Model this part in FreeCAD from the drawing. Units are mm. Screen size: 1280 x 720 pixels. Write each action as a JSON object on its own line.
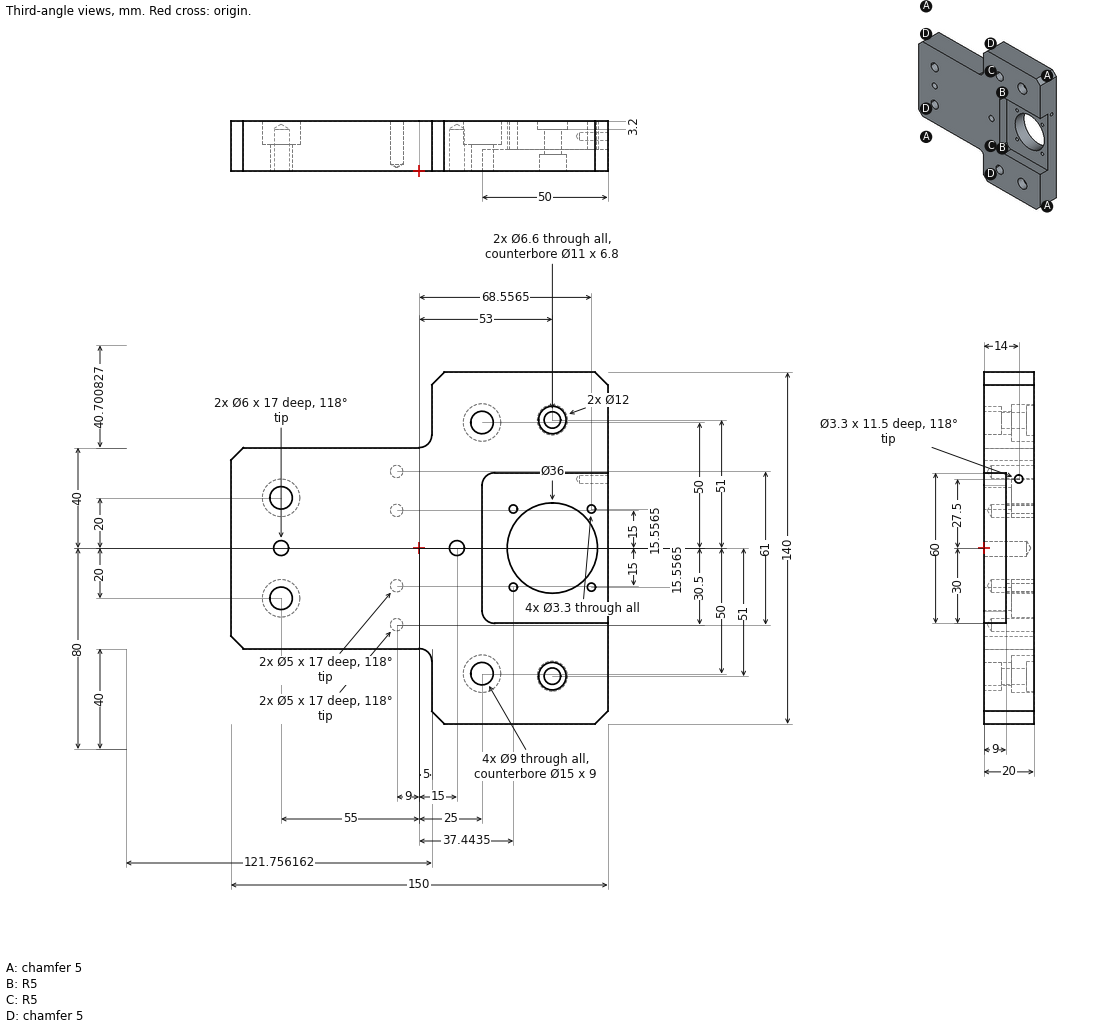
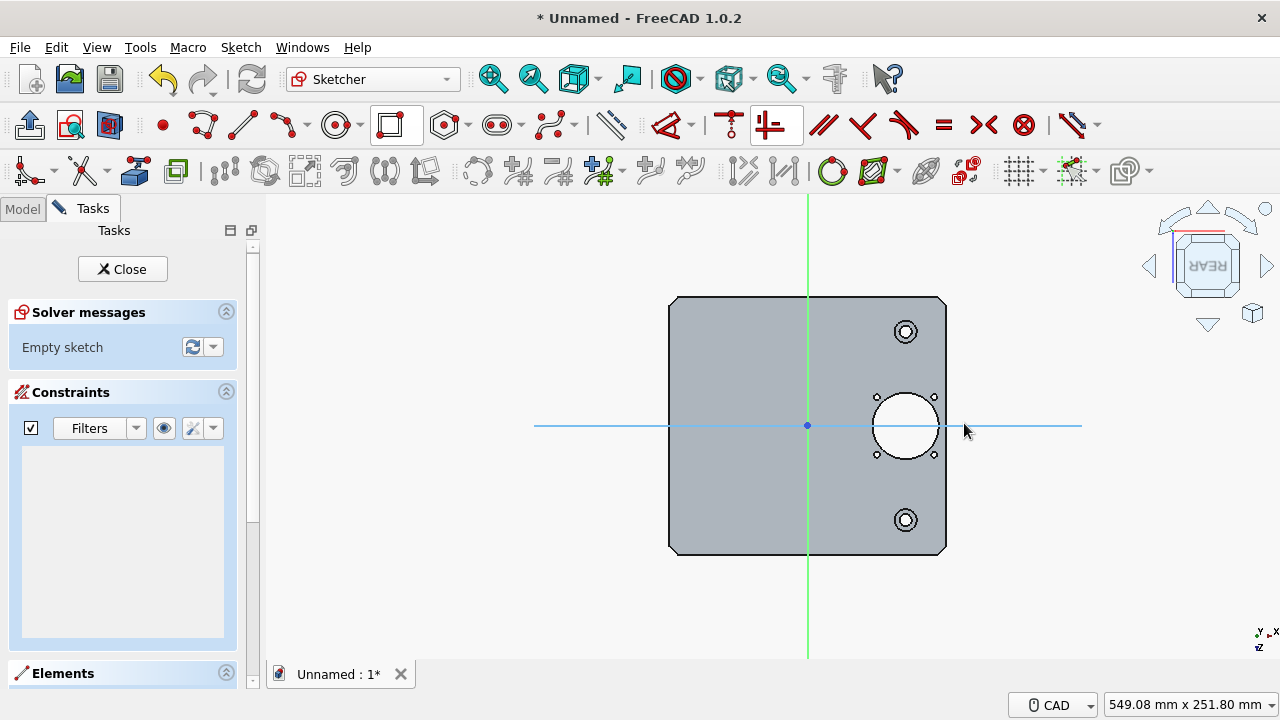
{"action": "left_click", "coordinate": [390, 126]}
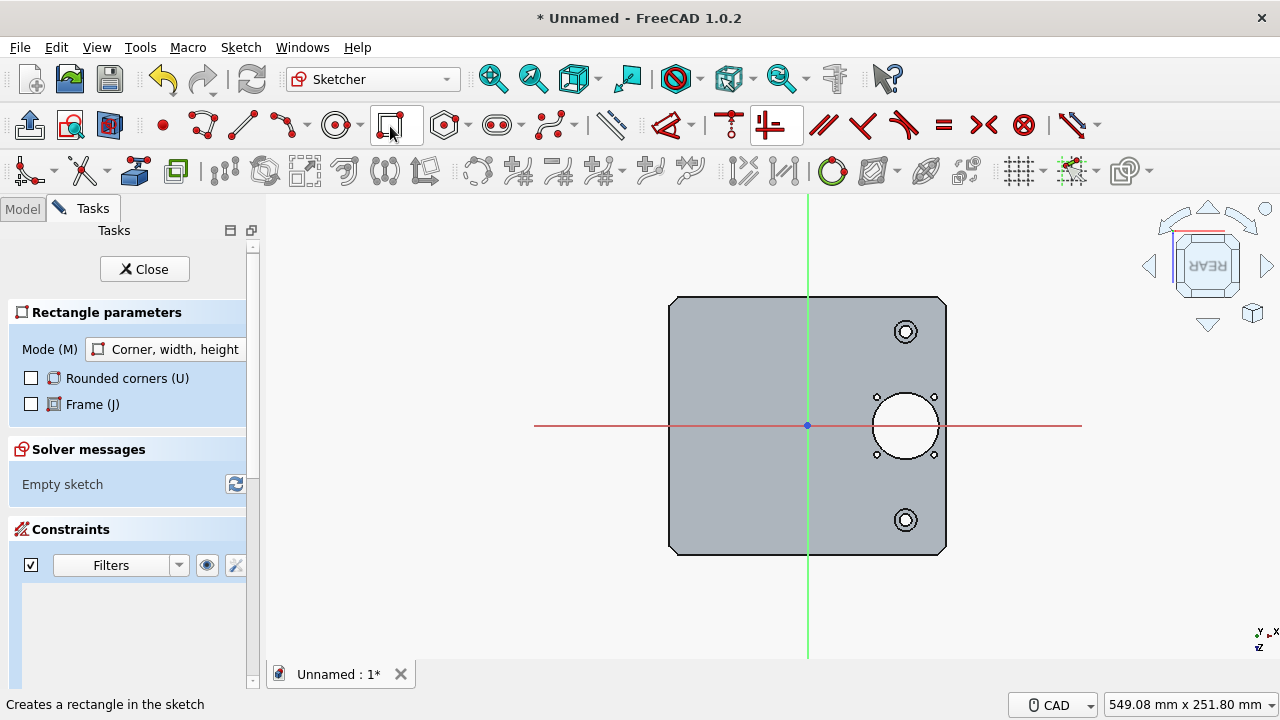
{"action": "left_click", "coordinate": [592, 278]}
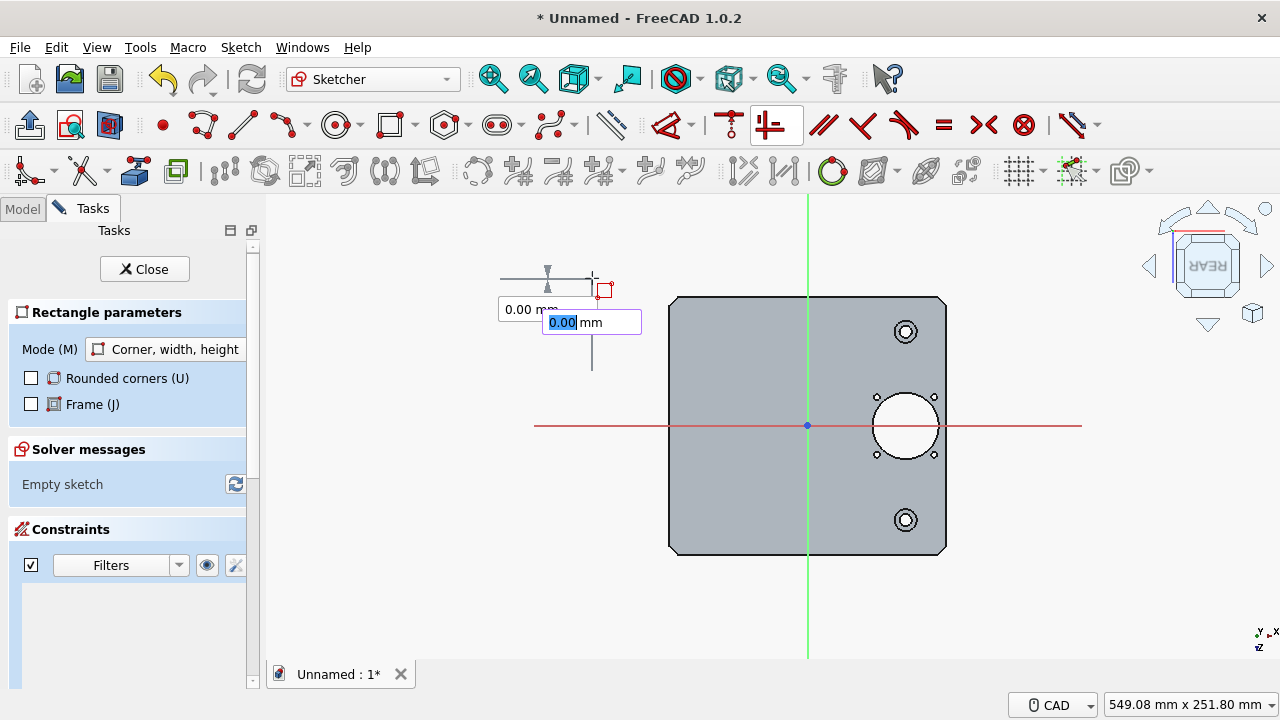
{"action": "scroll", "coordinate": [817, 352], "scroll_direction": "up", "scroll_amount": 3}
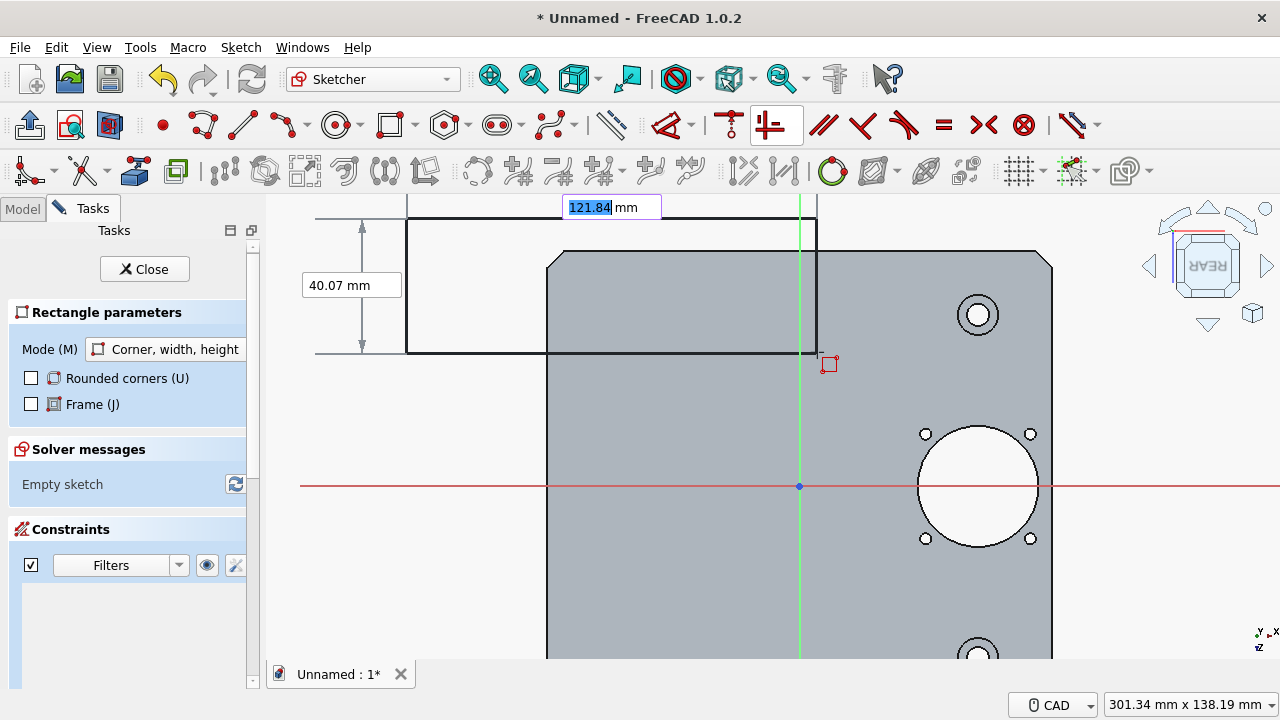
{"action": "left_click", "coordinate": [817, 352]}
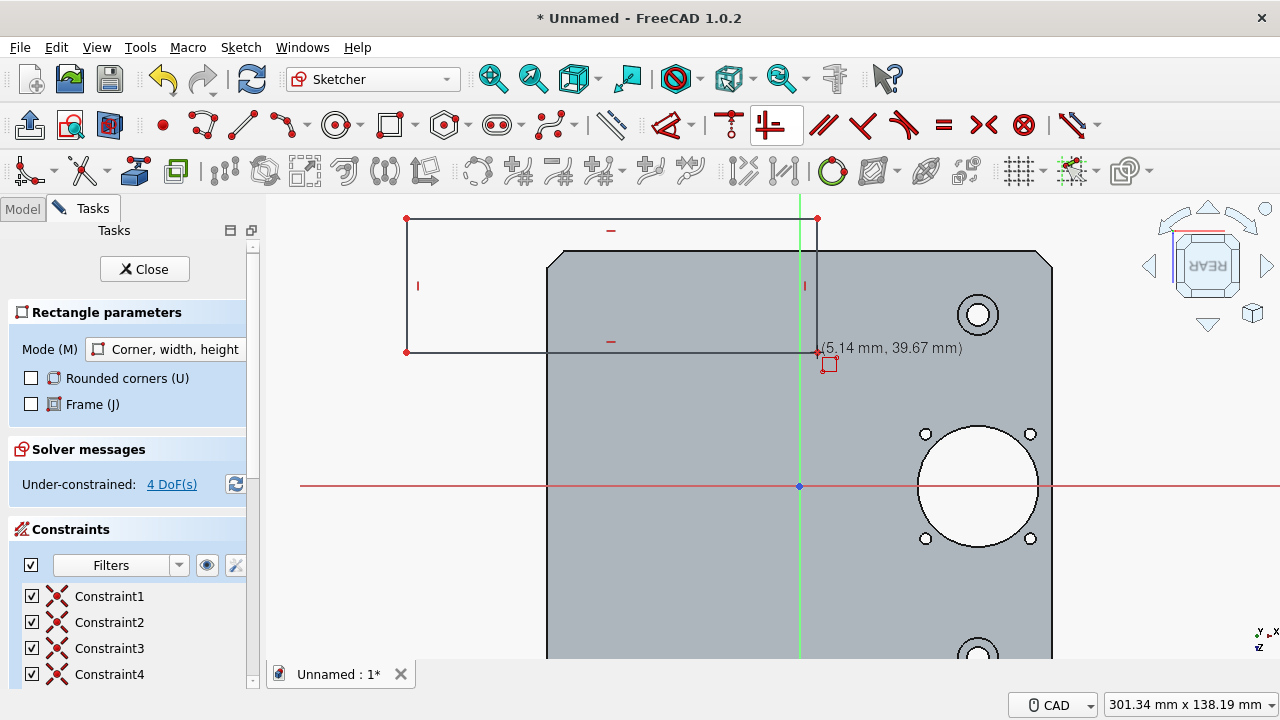
{"action": "left_click", "coordinate": [407, 621]}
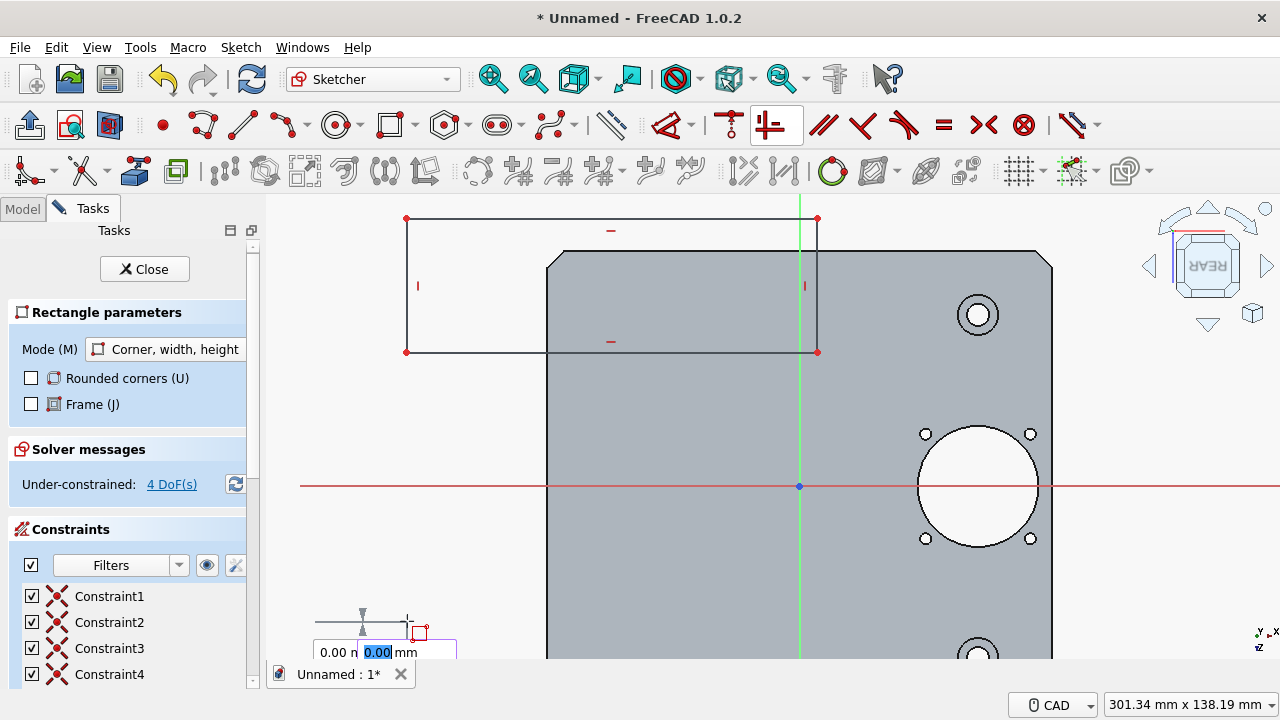
{"action": "scroll", "coordinate": [817, 352], "scroll_direction": "down", "scroll_amount": 3}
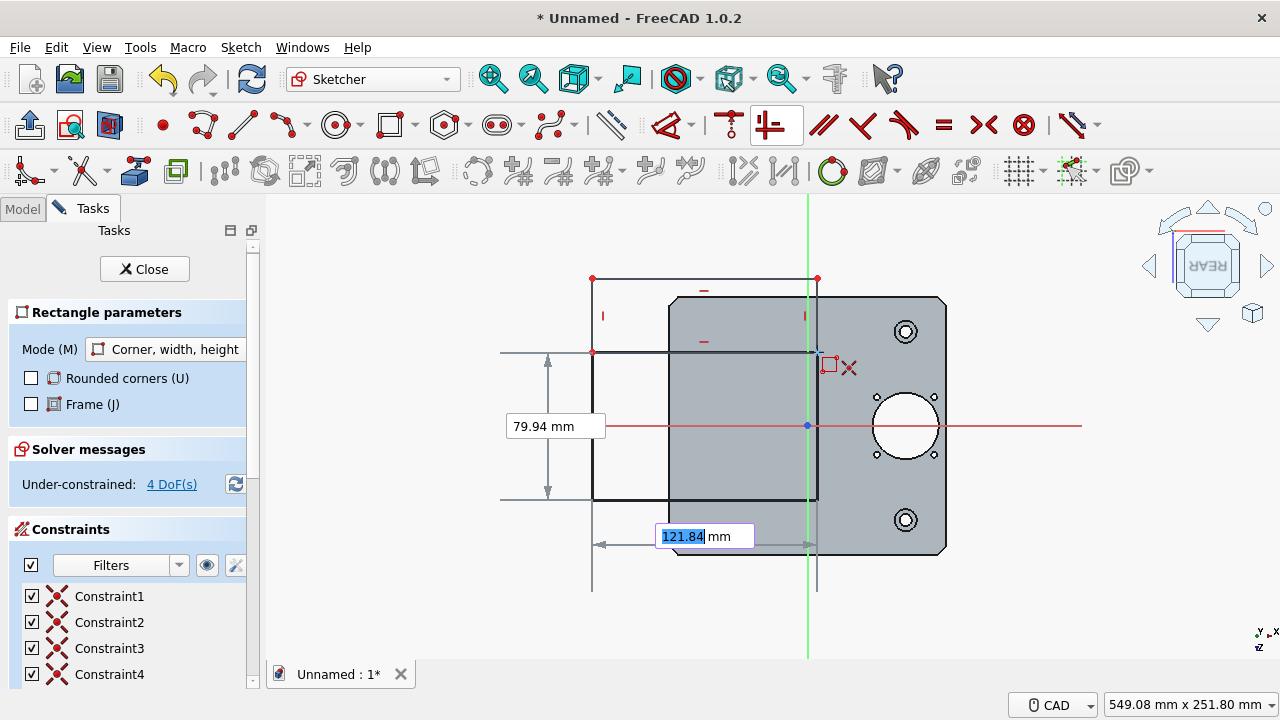
{"action": "scroll", "coordinate": [817, 575], "scroll_direction": "up", "scroll_amount": 3}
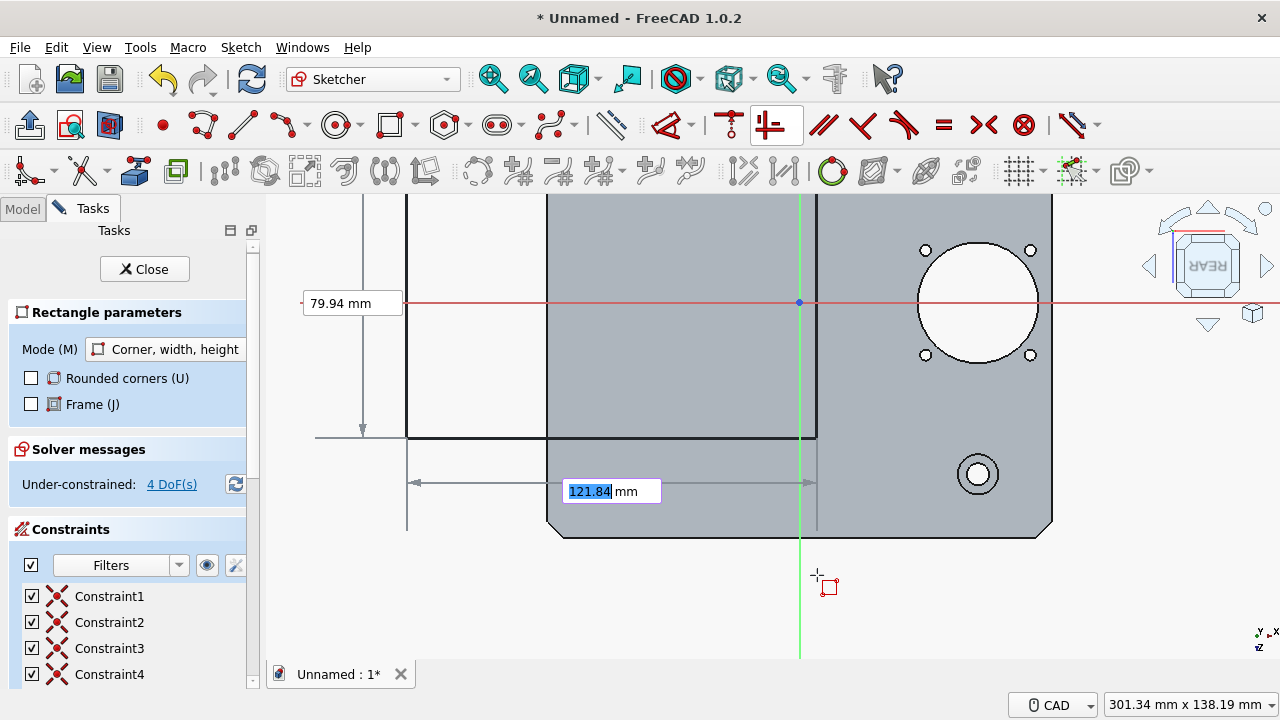
{"action": "left_click", "coordinate": [817, 574]}
{"action": "key", "text": "Escape"}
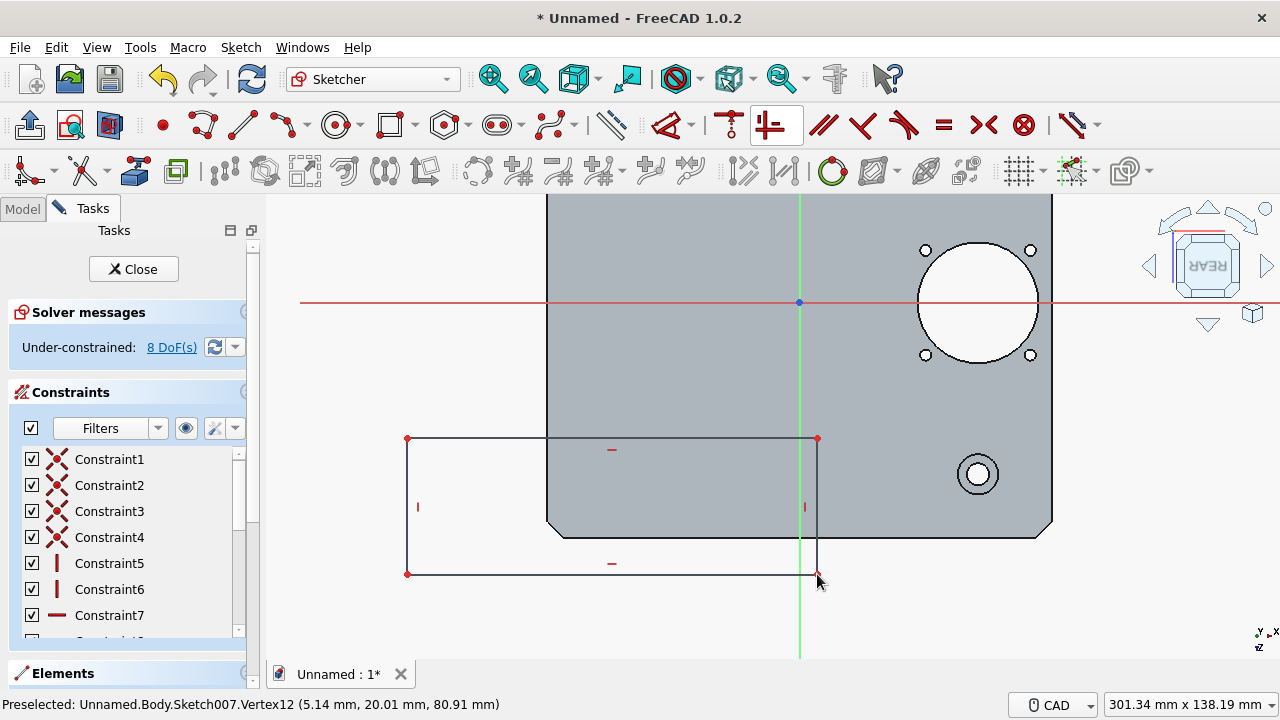
{"action": "left_click", "coordinate": [666, 126]}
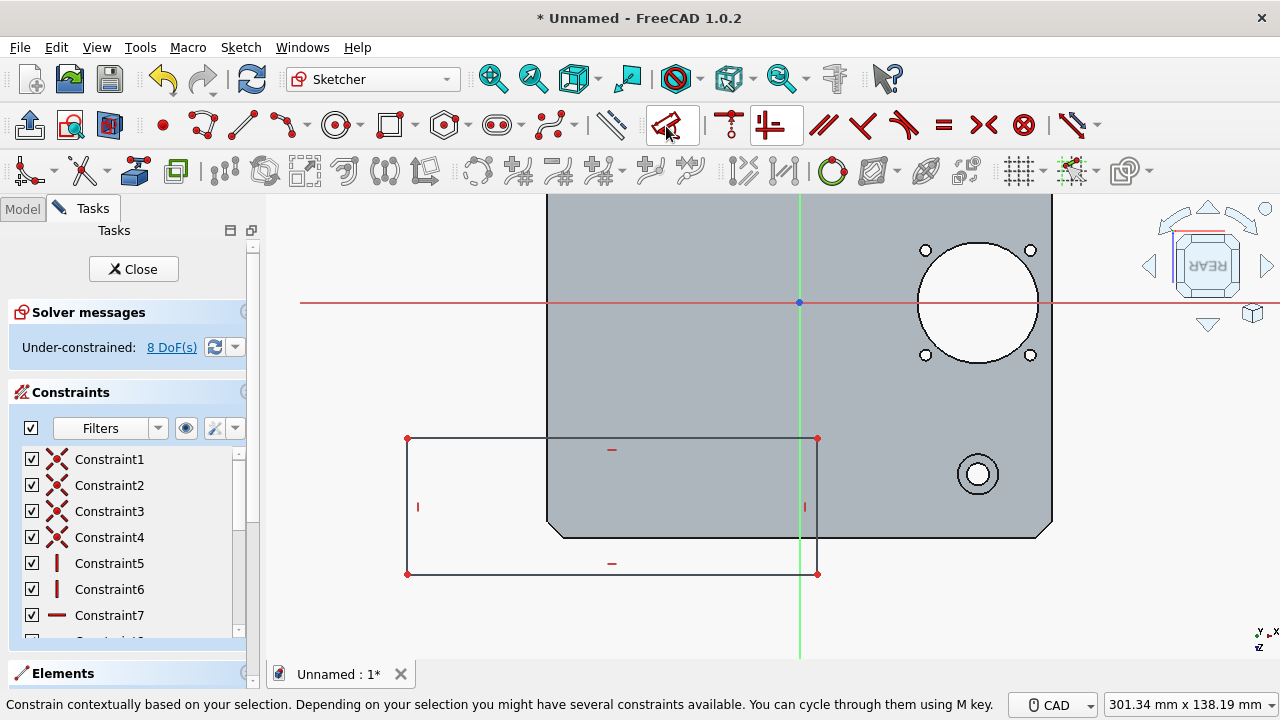
{"action": "scroll", "coordinate": [817, 576], "scroll_direction": "down", "scroll_amount": 3}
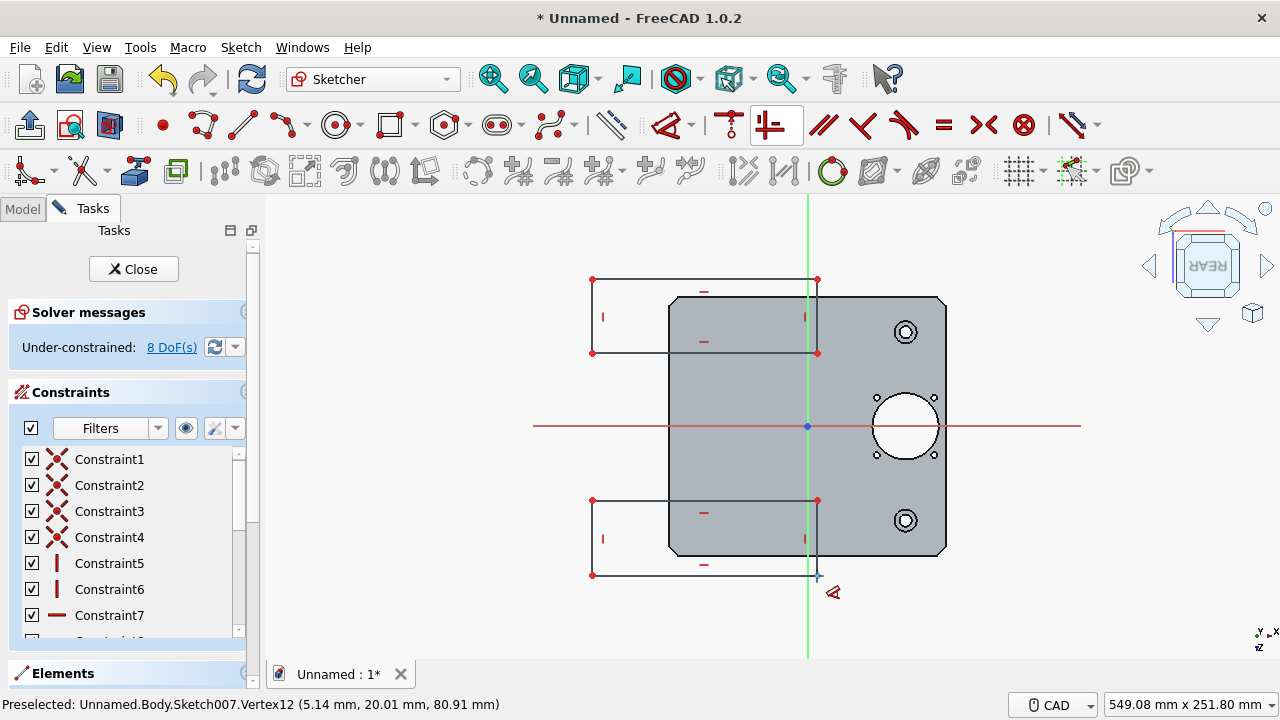
{"action": "left_click", "coordinate": [592, 302]}
{"action": "left_click", "coordinate": [558, 316]}